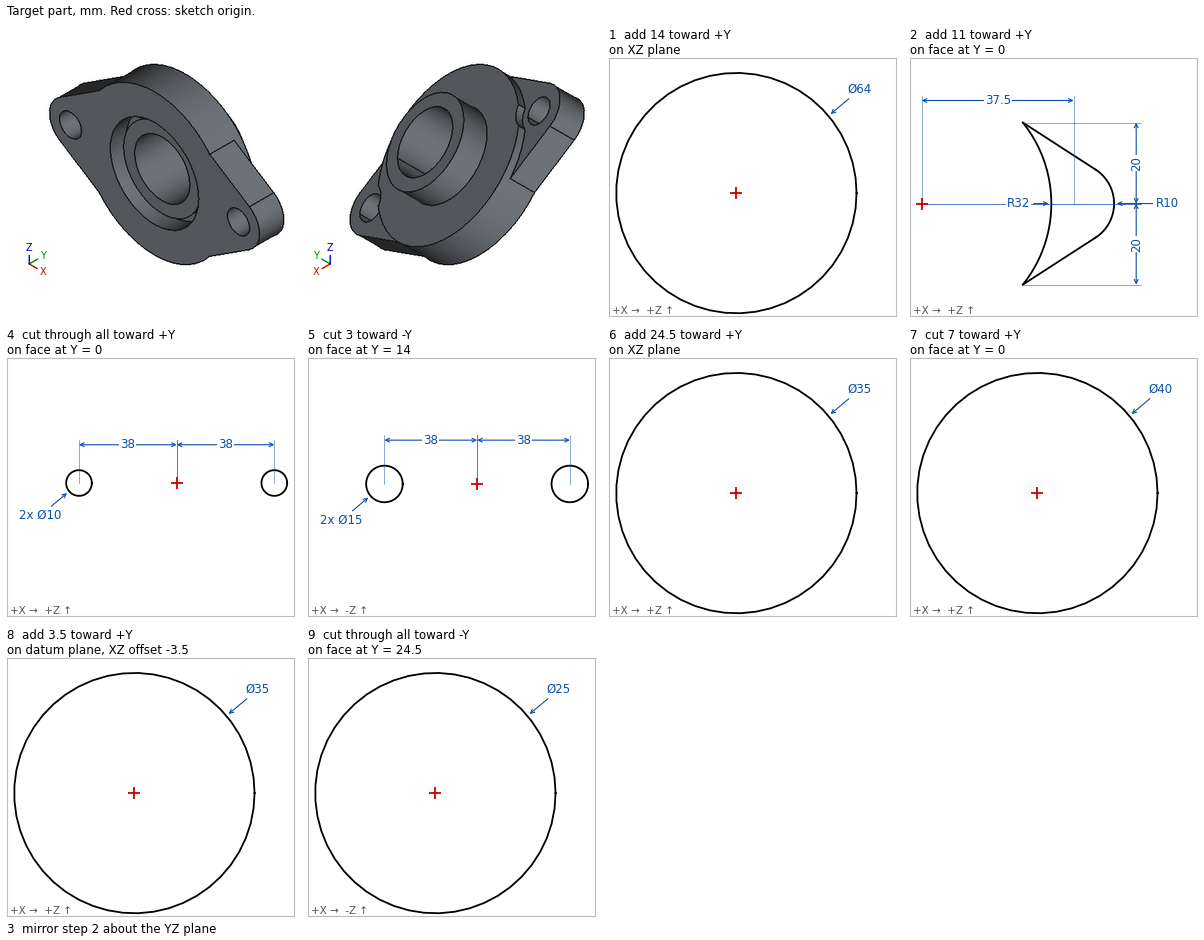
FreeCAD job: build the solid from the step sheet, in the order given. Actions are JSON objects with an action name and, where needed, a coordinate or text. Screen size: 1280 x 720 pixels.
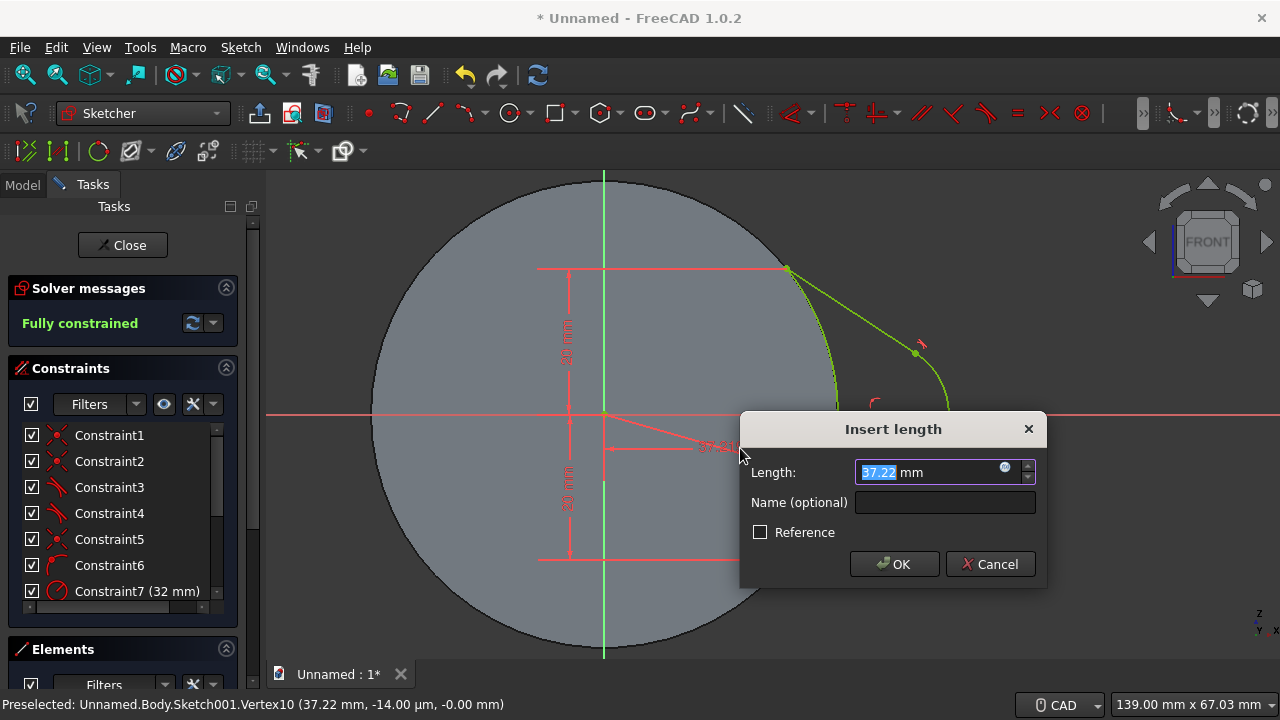
{"action": "type", "text": "37.5"}
{"action": "key", "text": "Return"}
{"action": "key", "text": "Escape"}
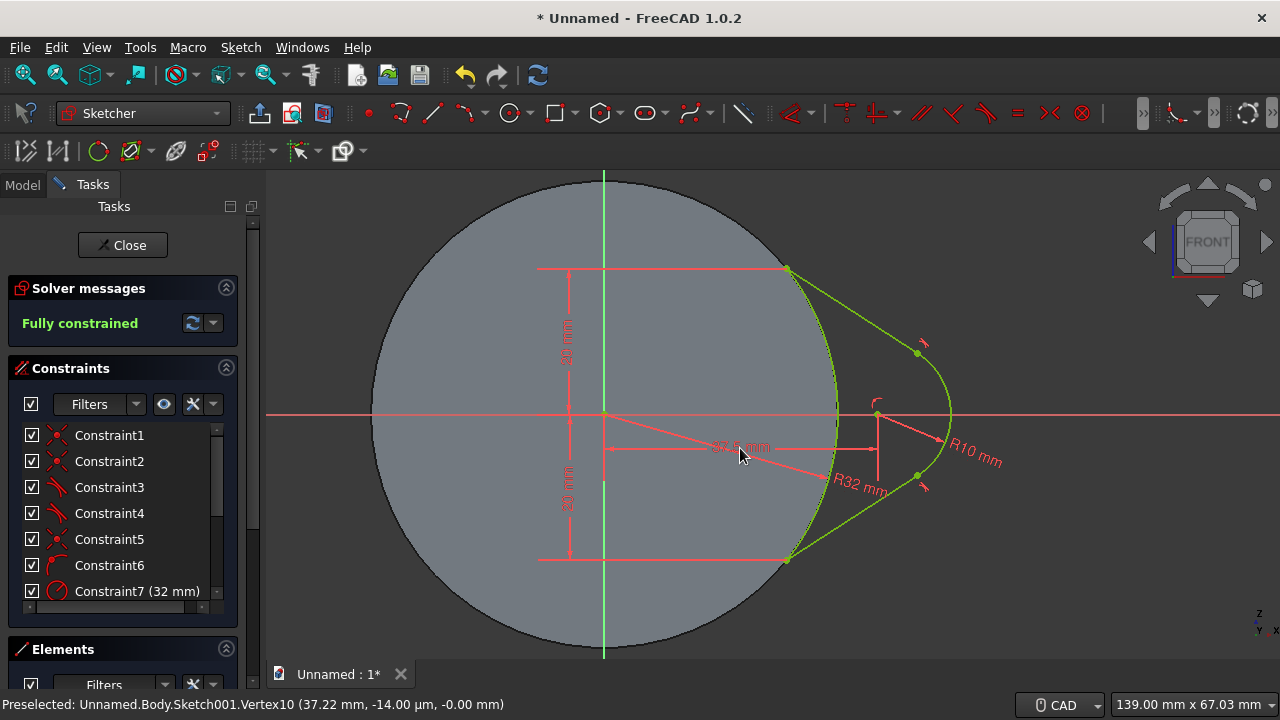
{"action": "left_click", "coordinate": [123, 245]}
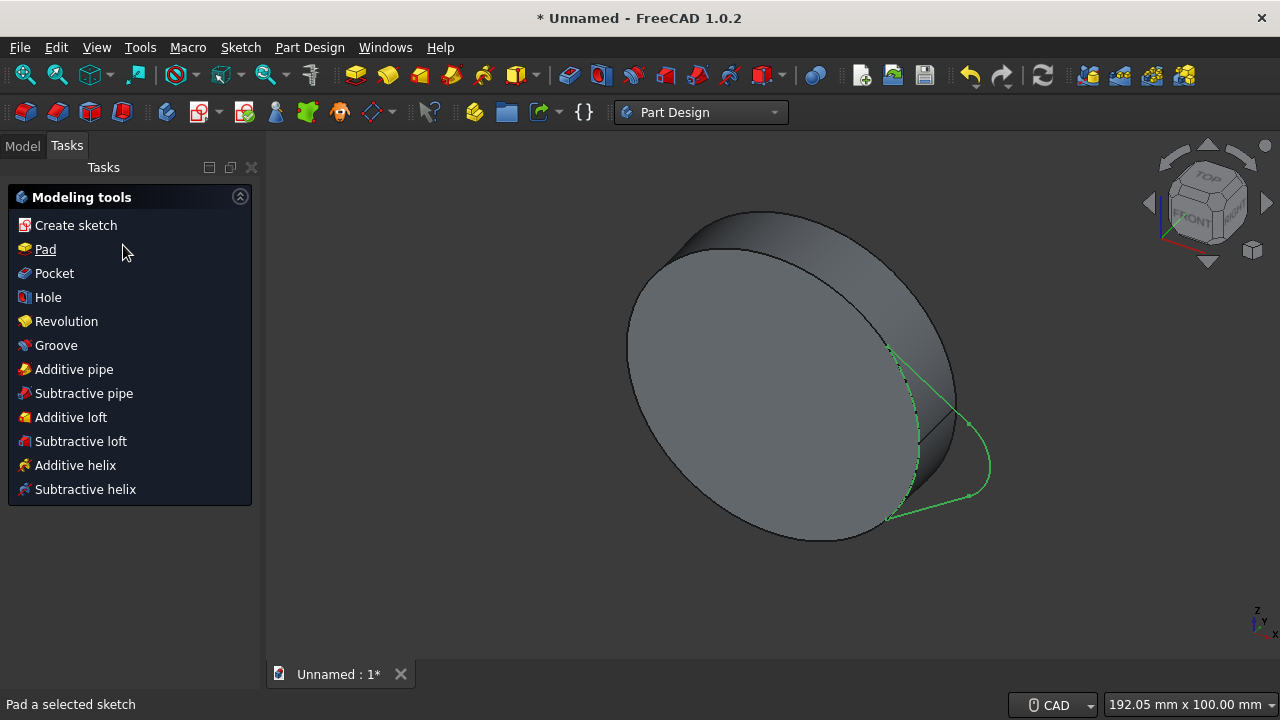
{"action": "left_click", "coordinate": [356, 76]}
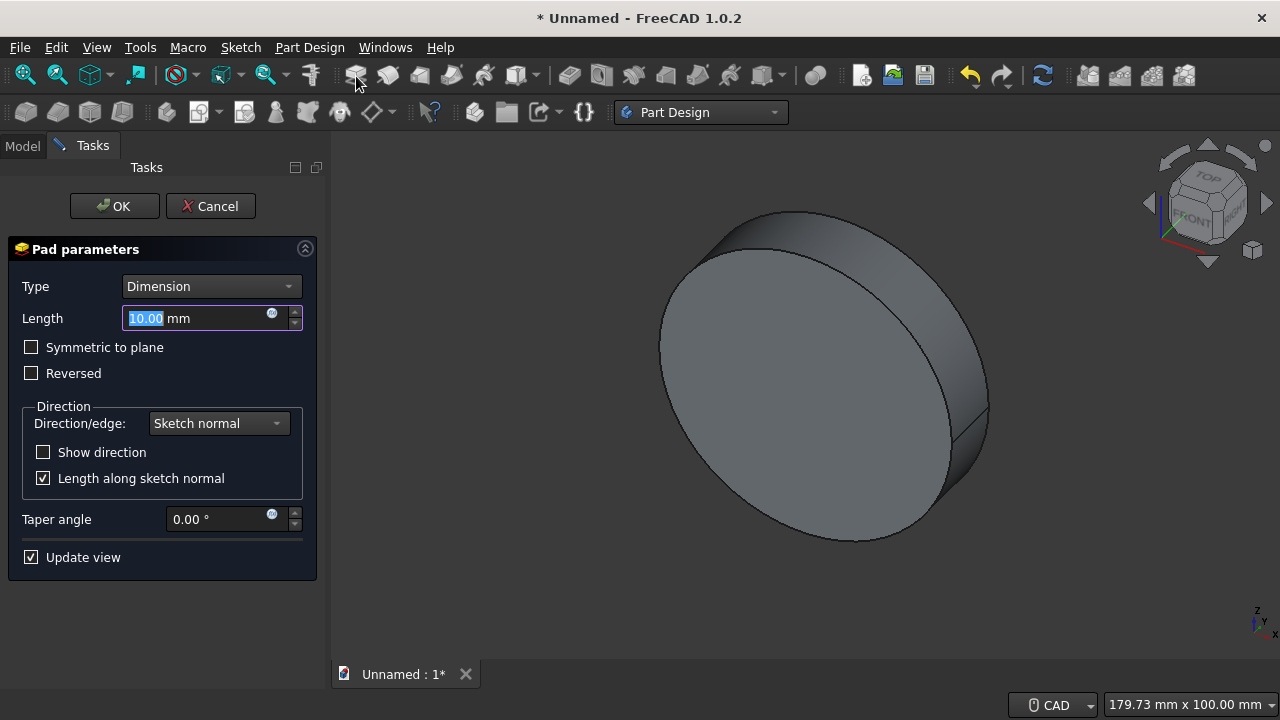
{"action": "type", "text": "11"}
{"action": "key", "text": "Tab"}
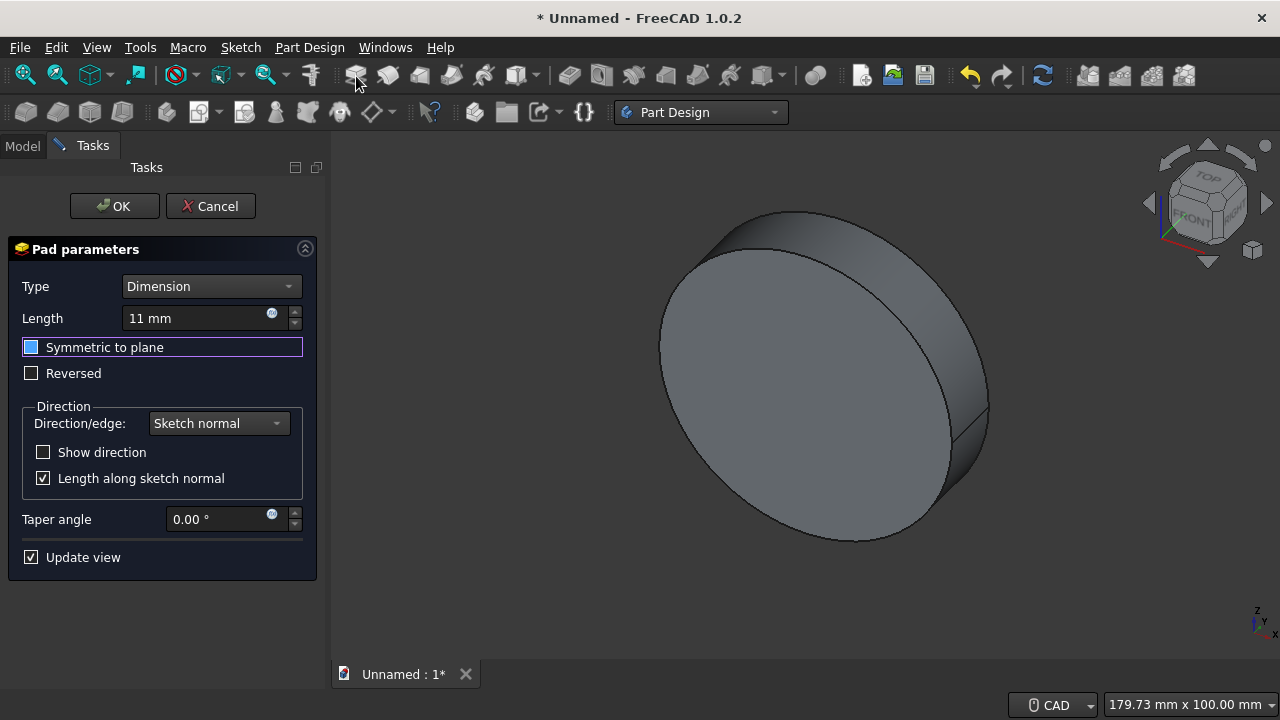
{"action": "left_click", "coordinate": [30, 373]}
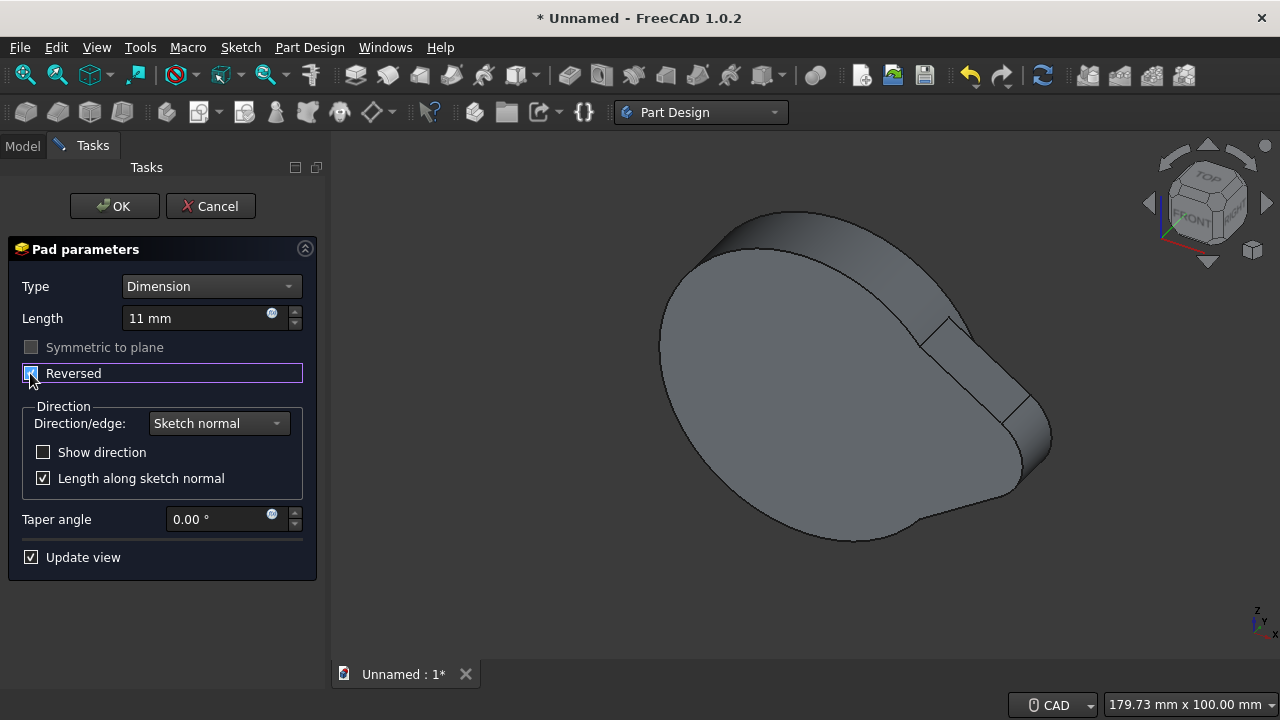
{"action": "left_click", "coordinate": [115, 206]}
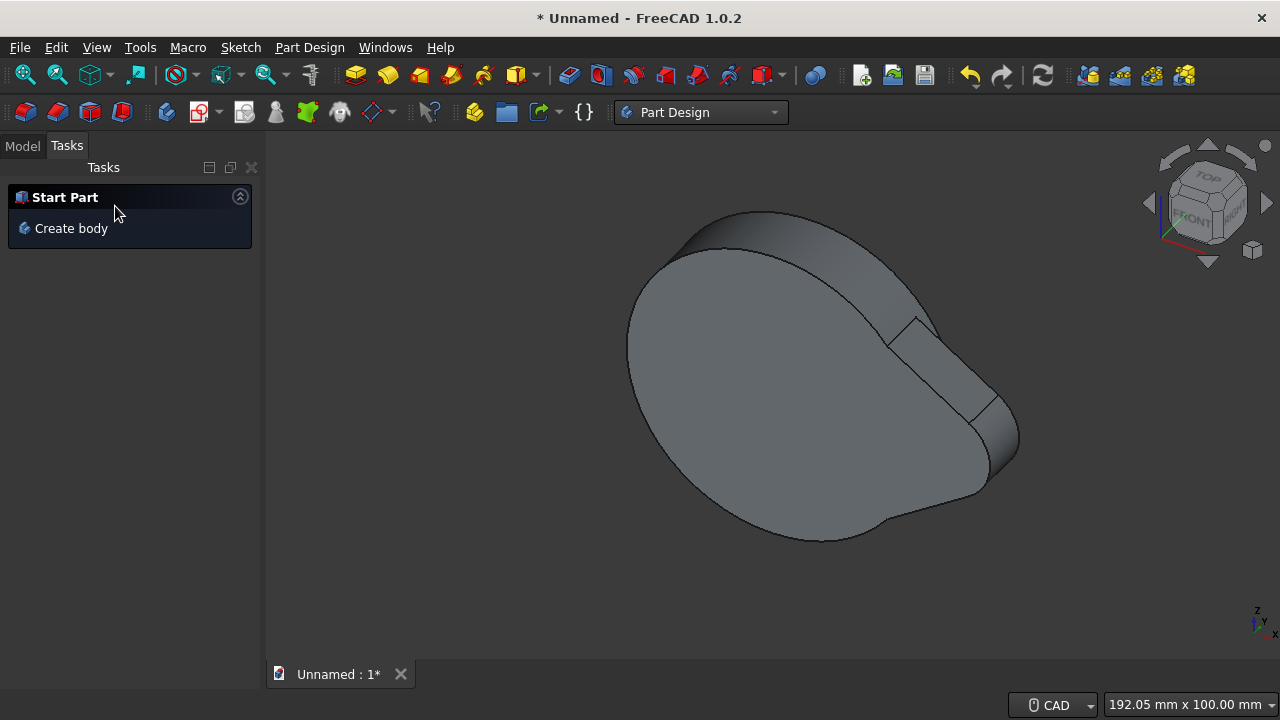
{"action": "left_click", "coordinate": [23, 145]}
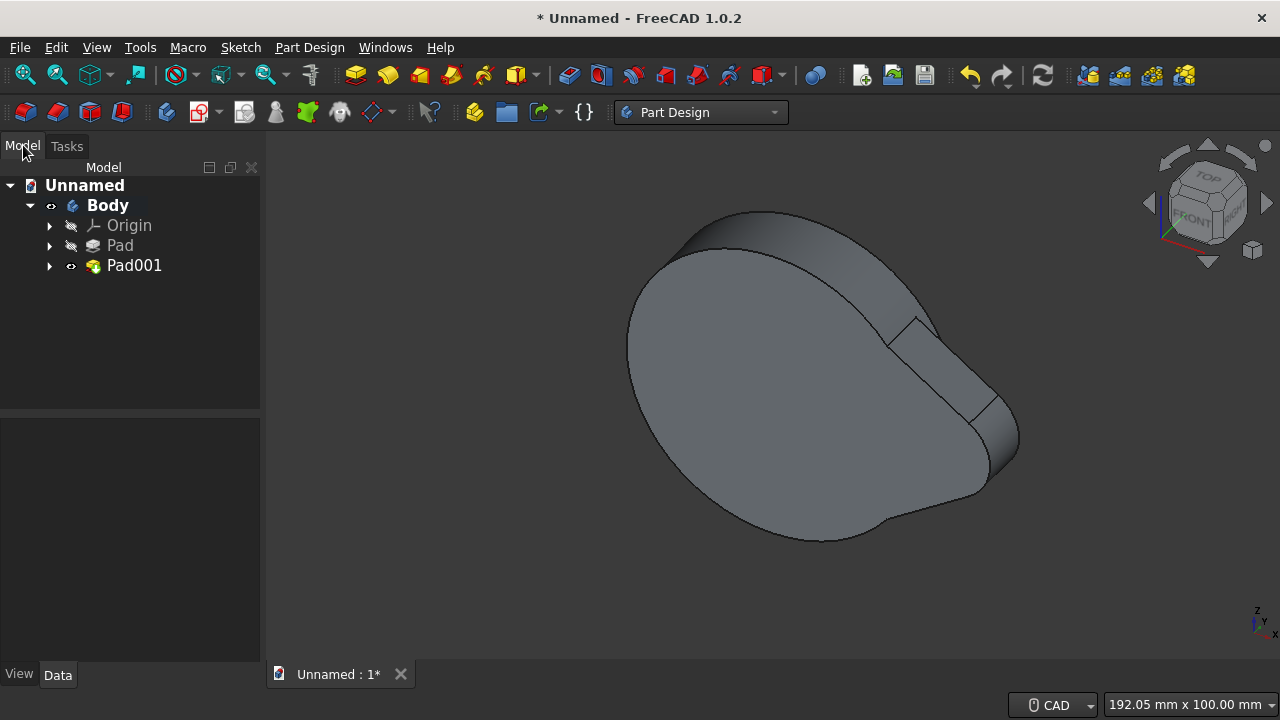
{"action": "left_click", "coordinate": [116, 266]}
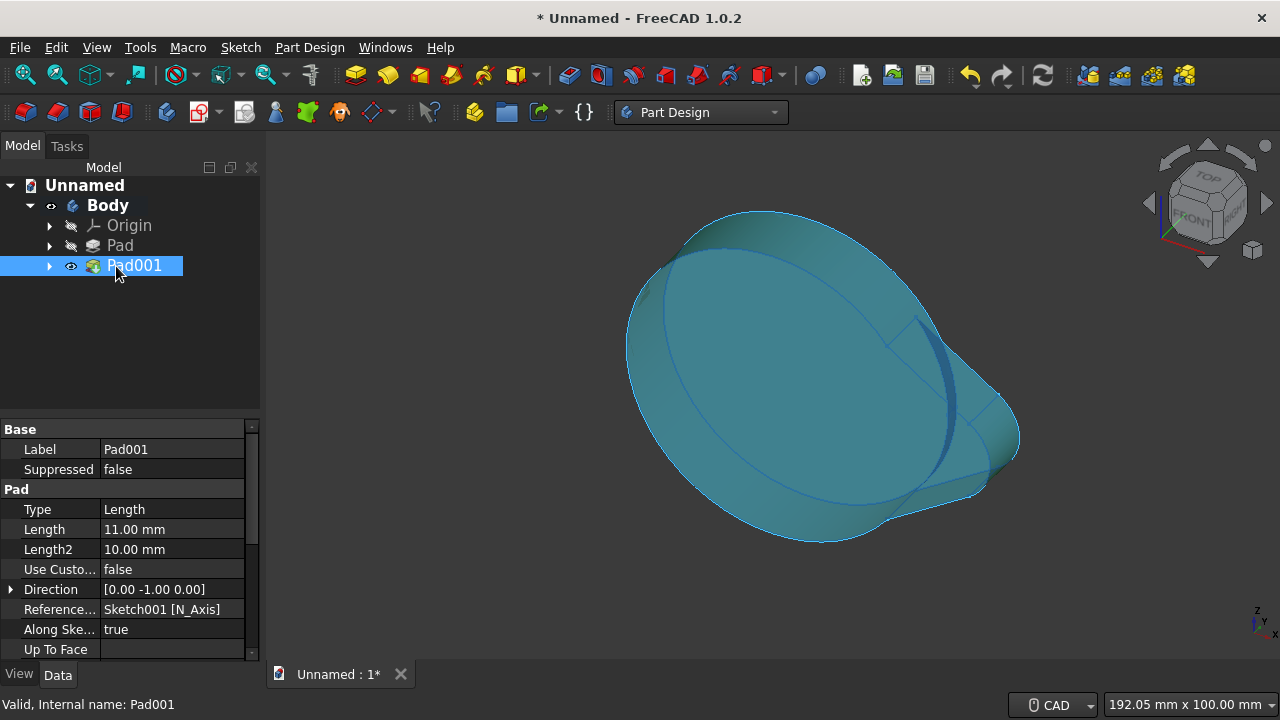
{"action": "left_click", "coordinate": [1088, 76]}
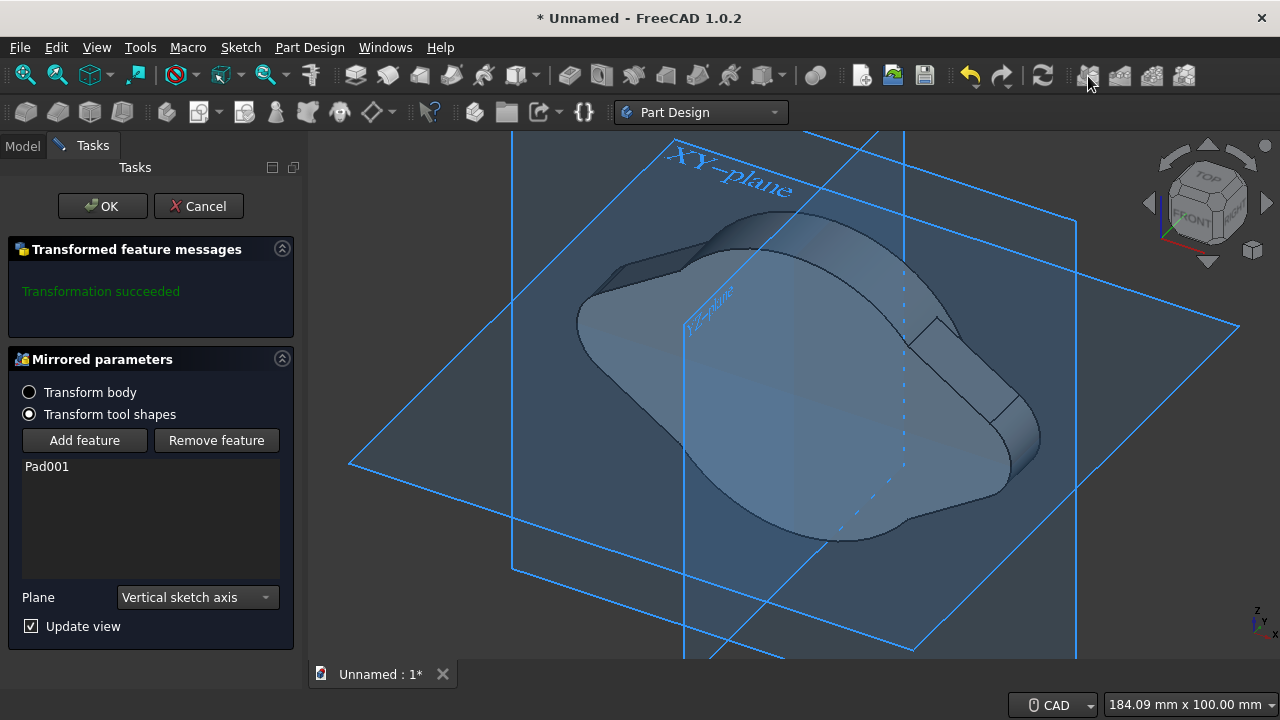
{"action": "left_click", "coordinate": [198, 598]}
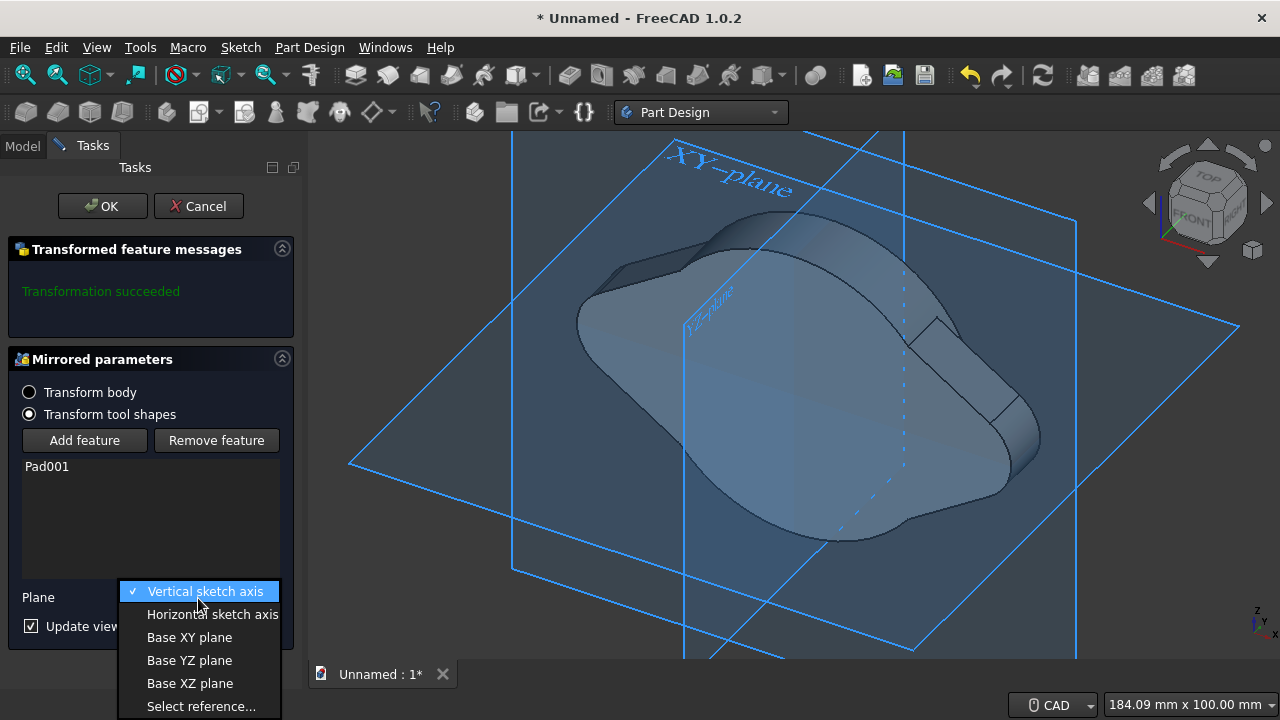
{"action": "left_click", "coordinate": [198, 660]}